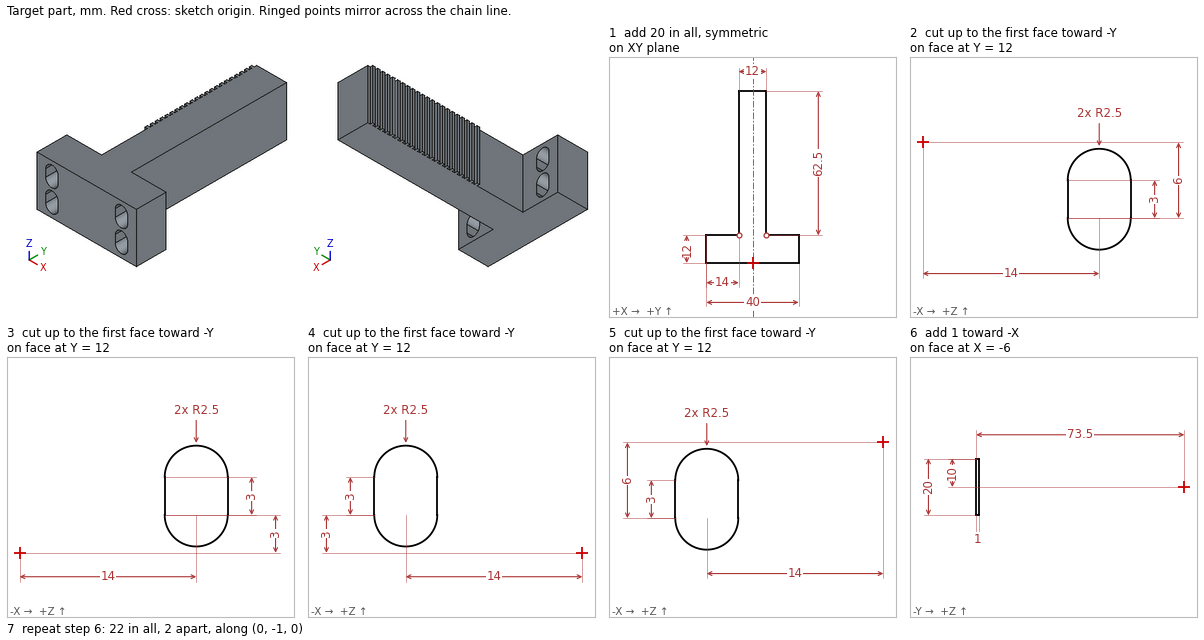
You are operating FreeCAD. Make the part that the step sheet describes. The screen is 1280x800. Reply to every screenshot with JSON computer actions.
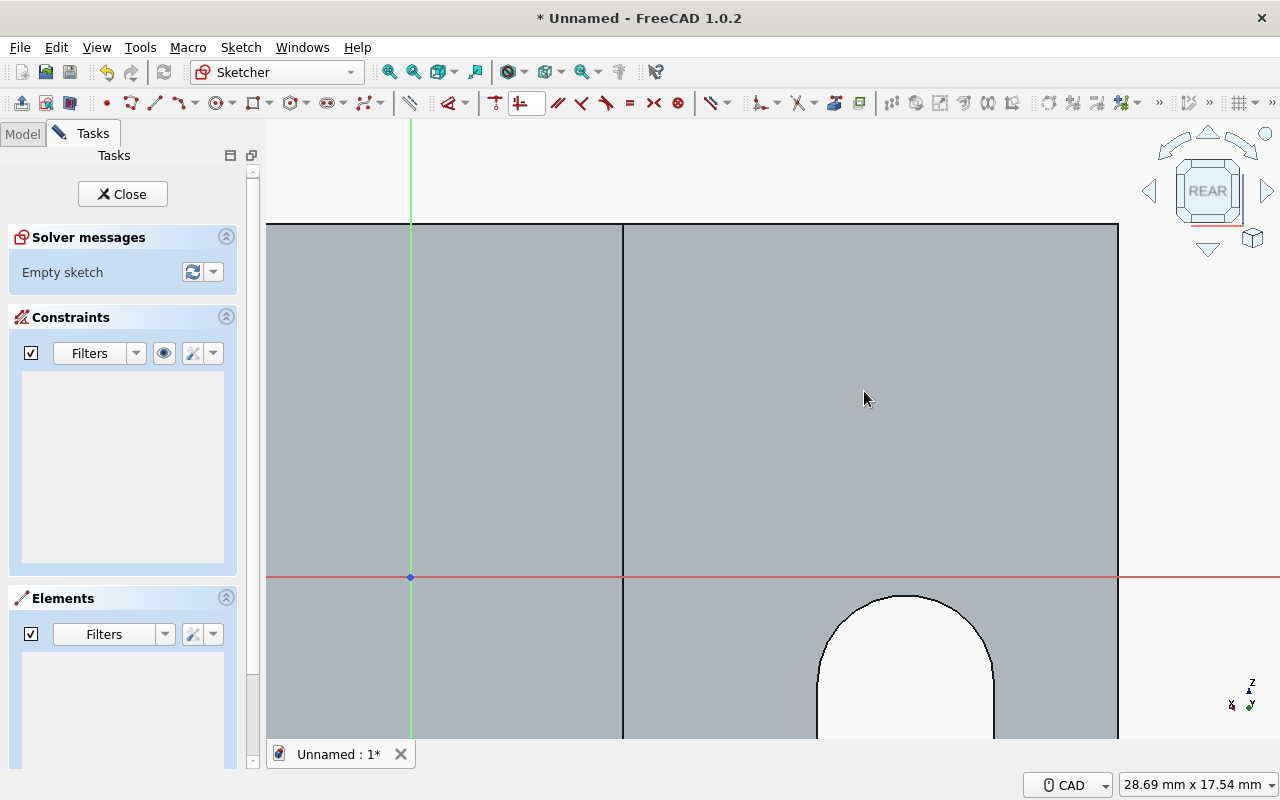
{"action": "left_click", "coordinate": [328, 104]}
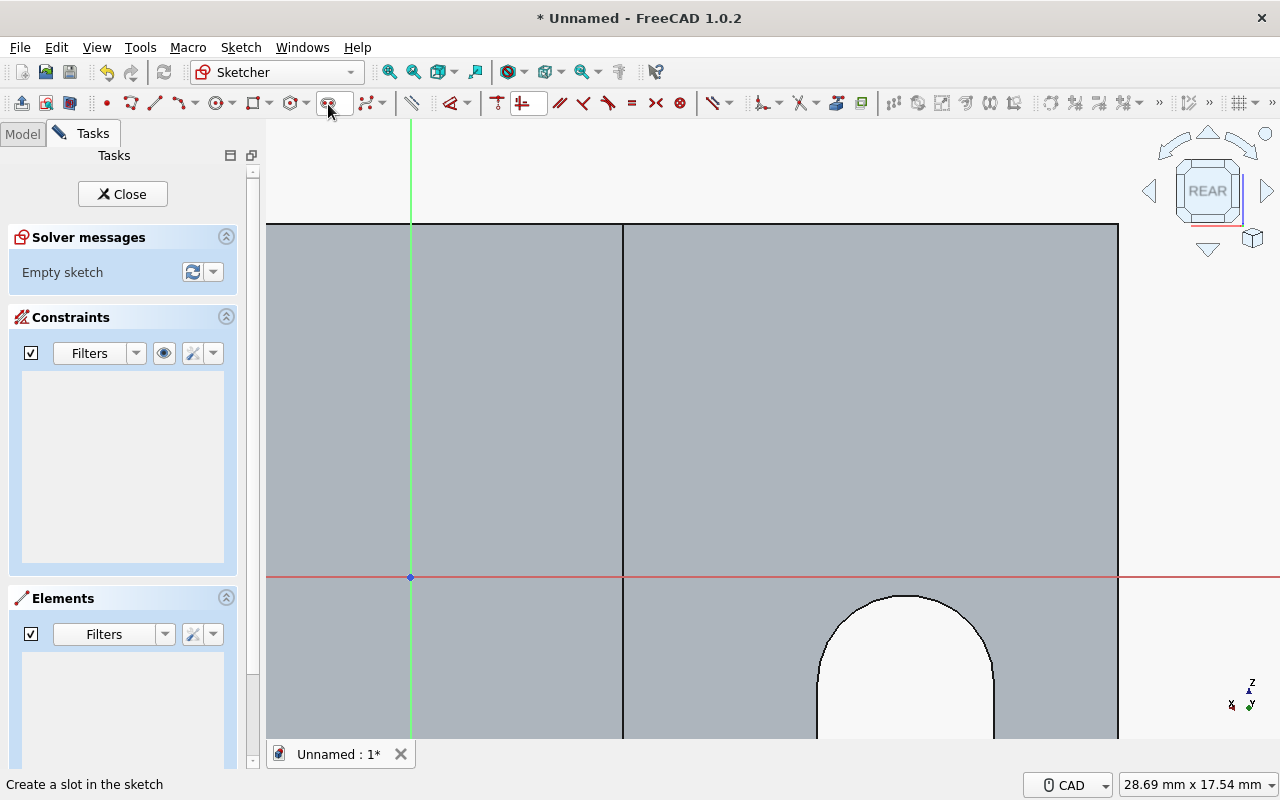
{"action": "left_click", "coordinate": [906, 471]}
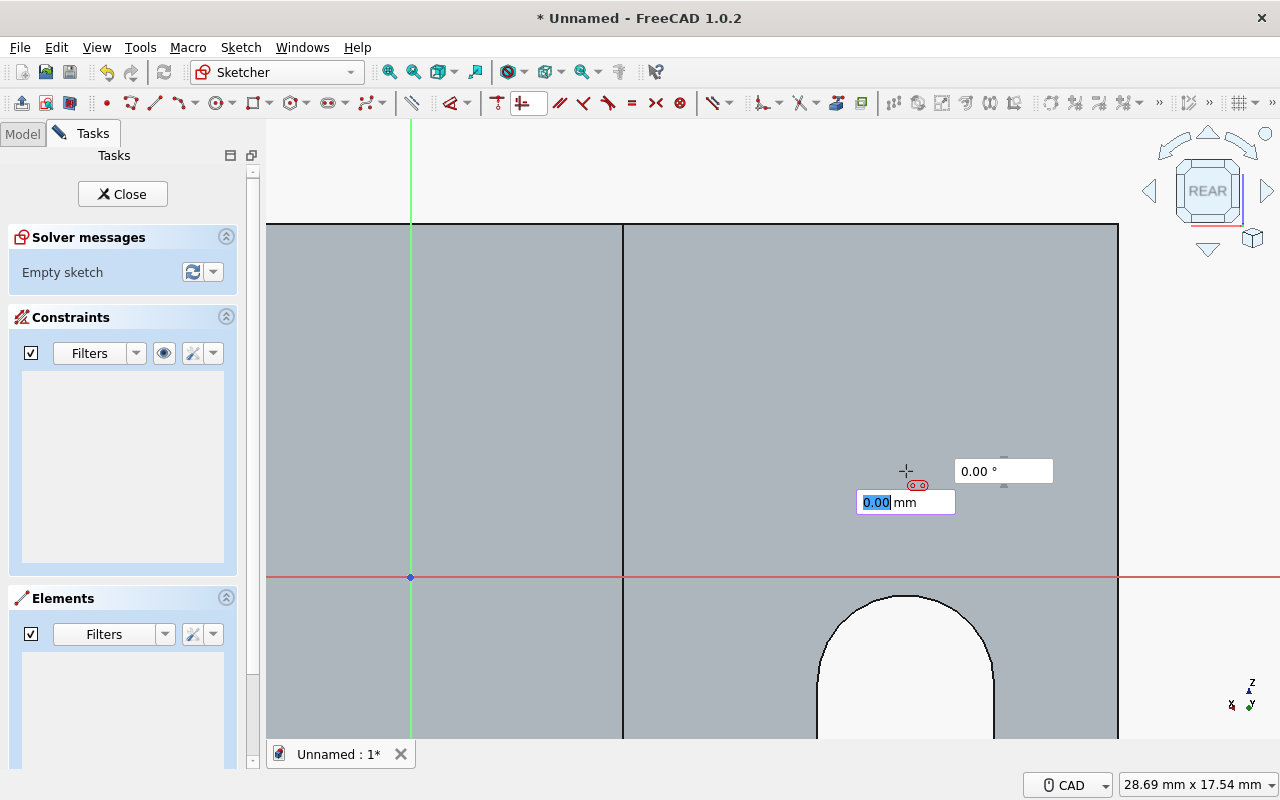
{"action": "left_click", "coordinate": [906, 365]}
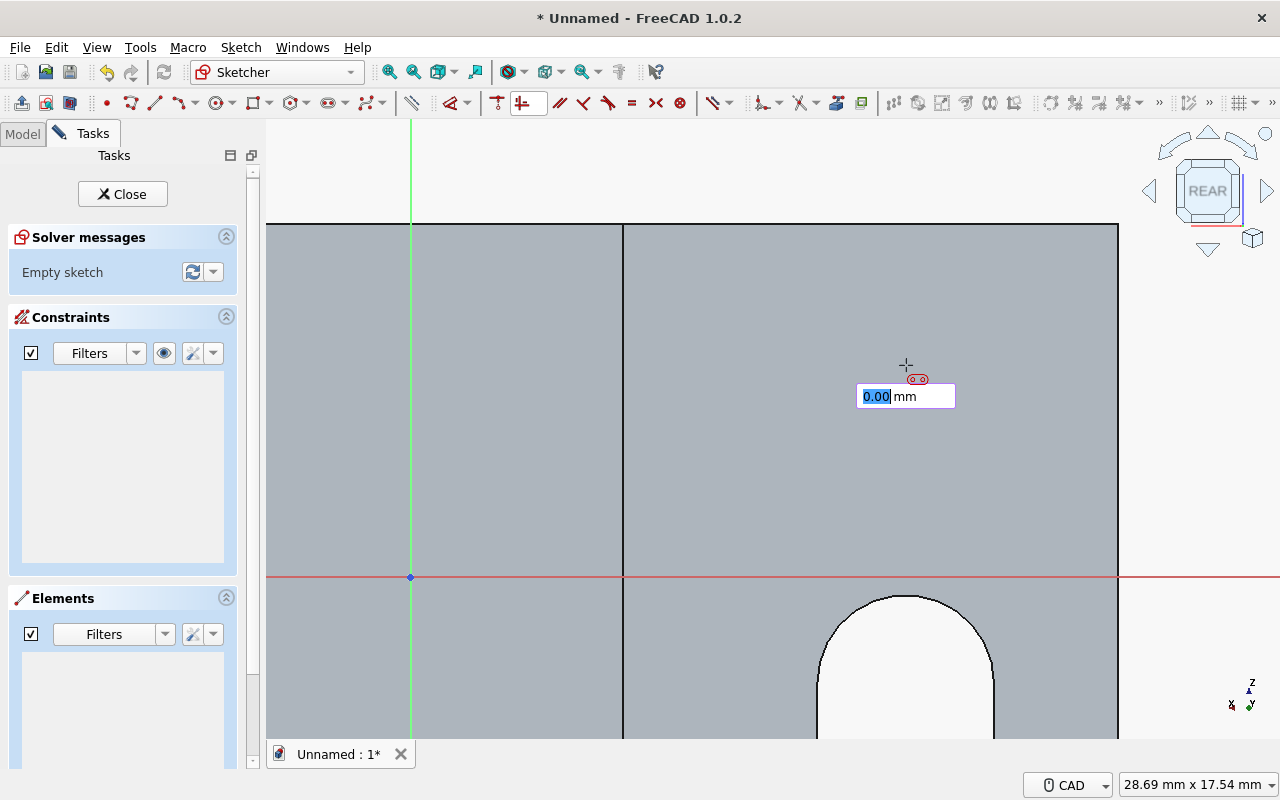
{"action": "left_click", "coordinate": [994, 418]}
{"action": "key", "text": "Escape"}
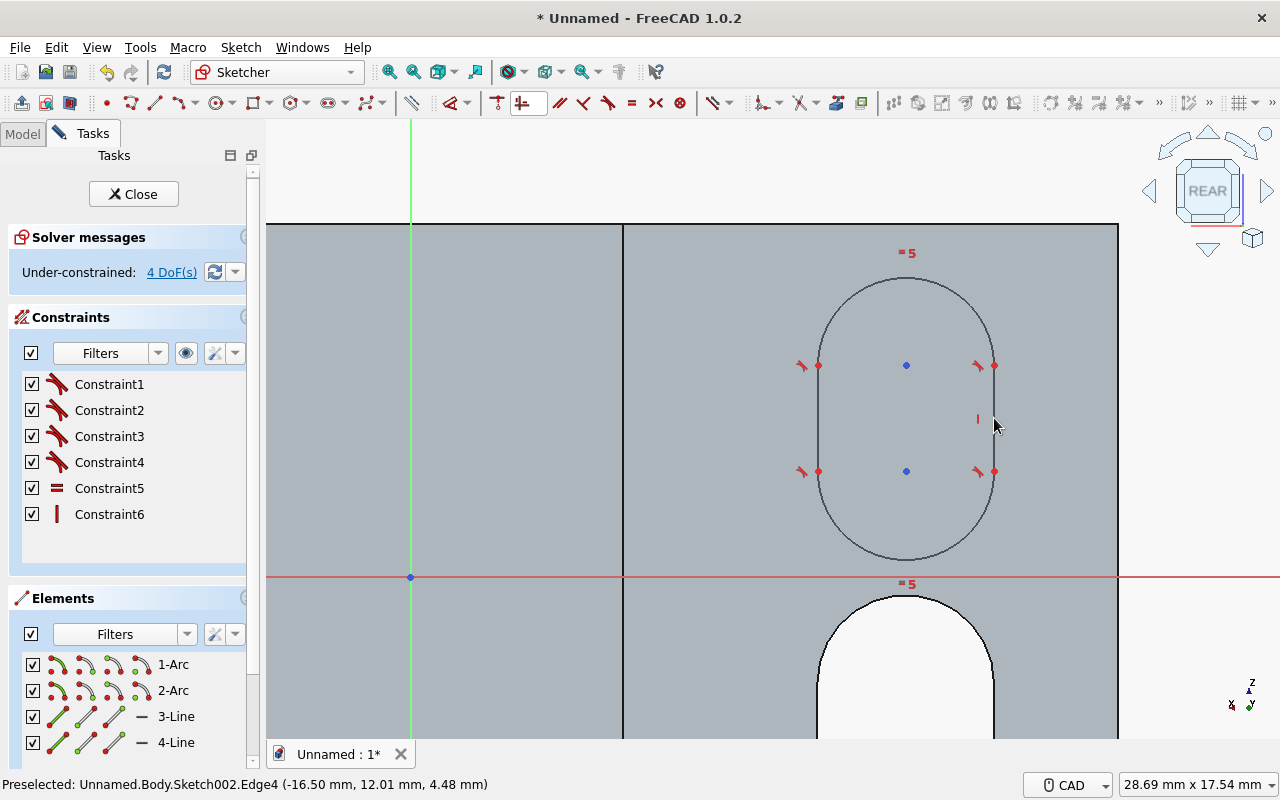
{"action": "left_click", "coordinate": [450, 104]}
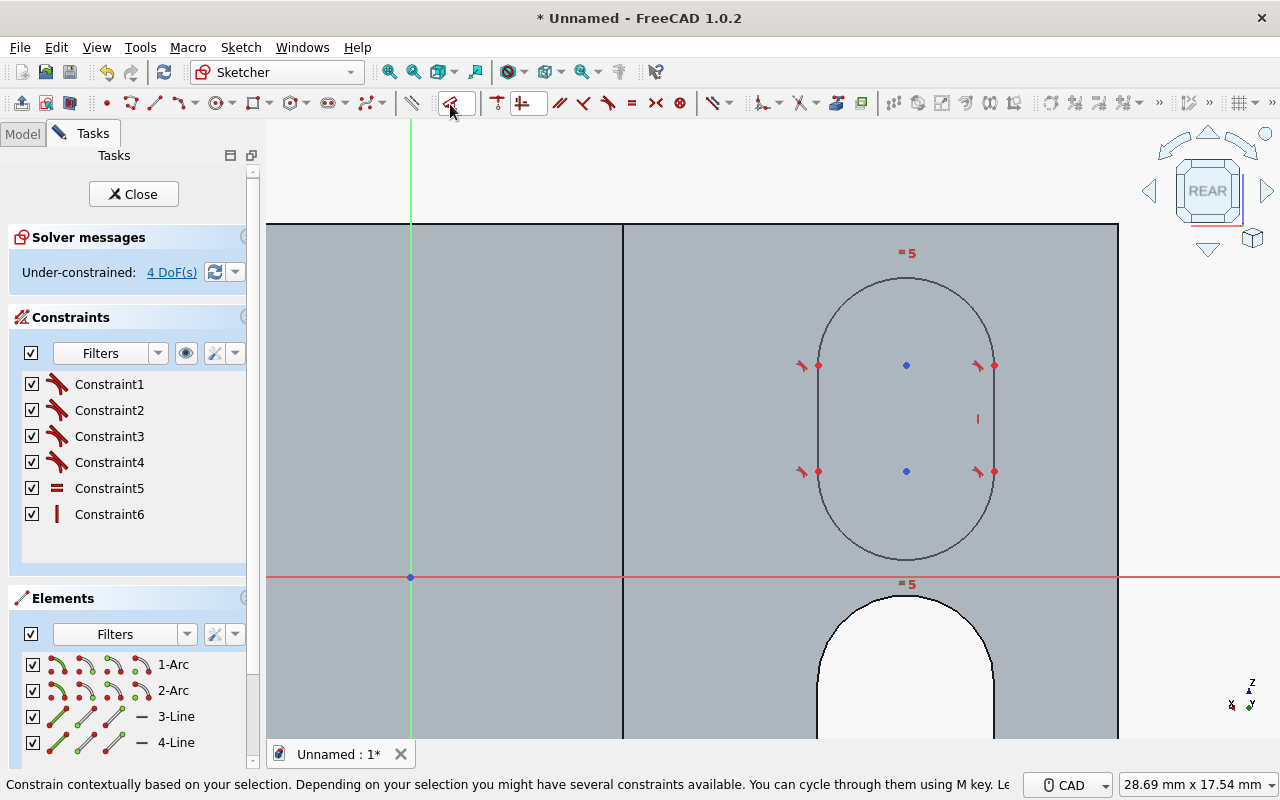
{"action": "left_click", "coordinate": [854, 543]}
{"action": "left_click", "coordinate": [797, 523]}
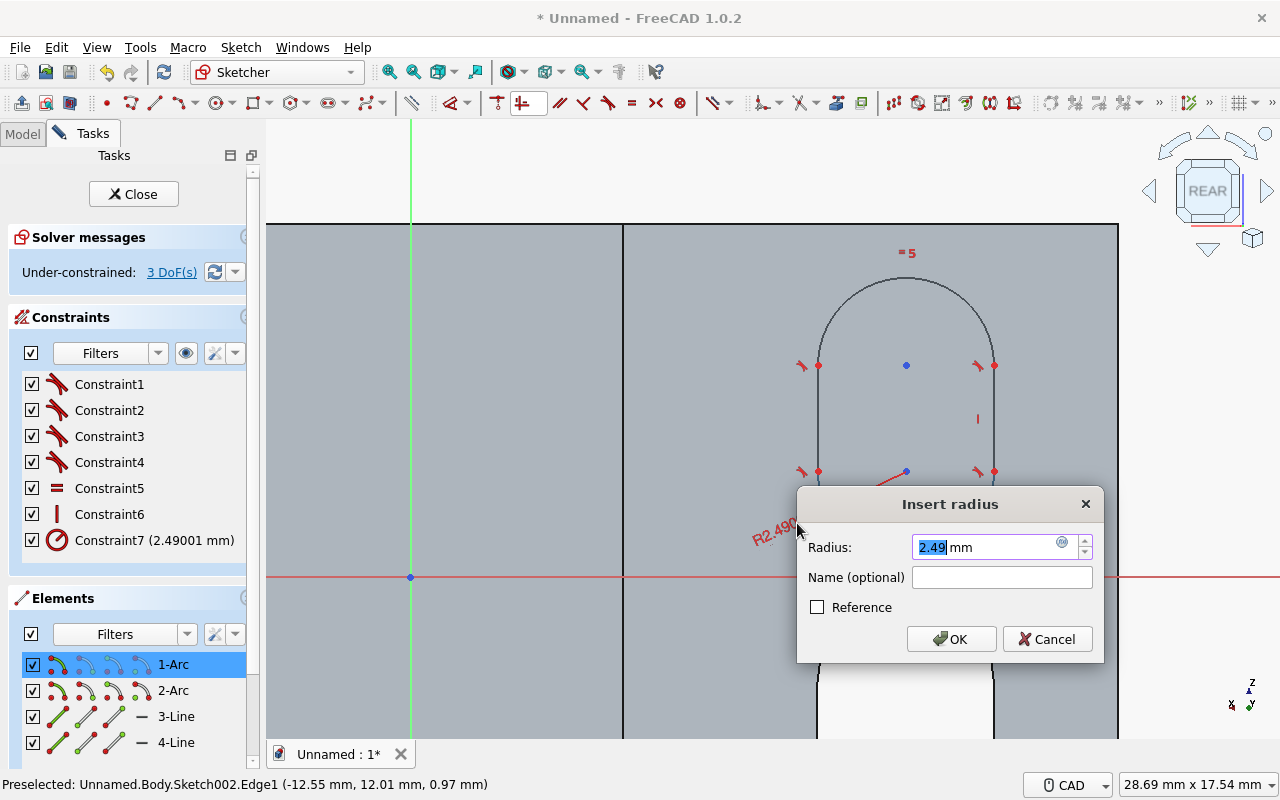
{"action": "type", "text": "2.5"}
{"action": "key", "text": "Return"}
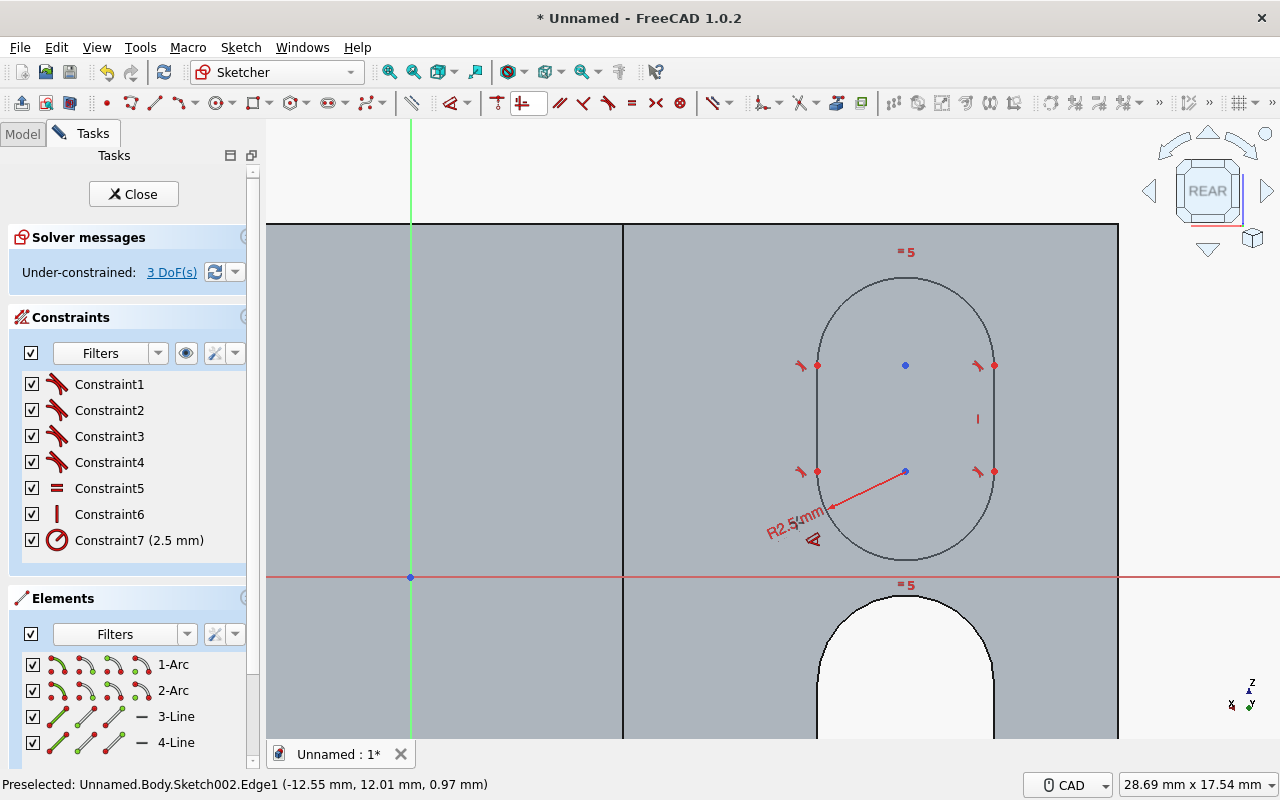
{"action": "left_click", "coordinate": [817, 440]}
{"action": "left_click", "coordinate": [851, 419]}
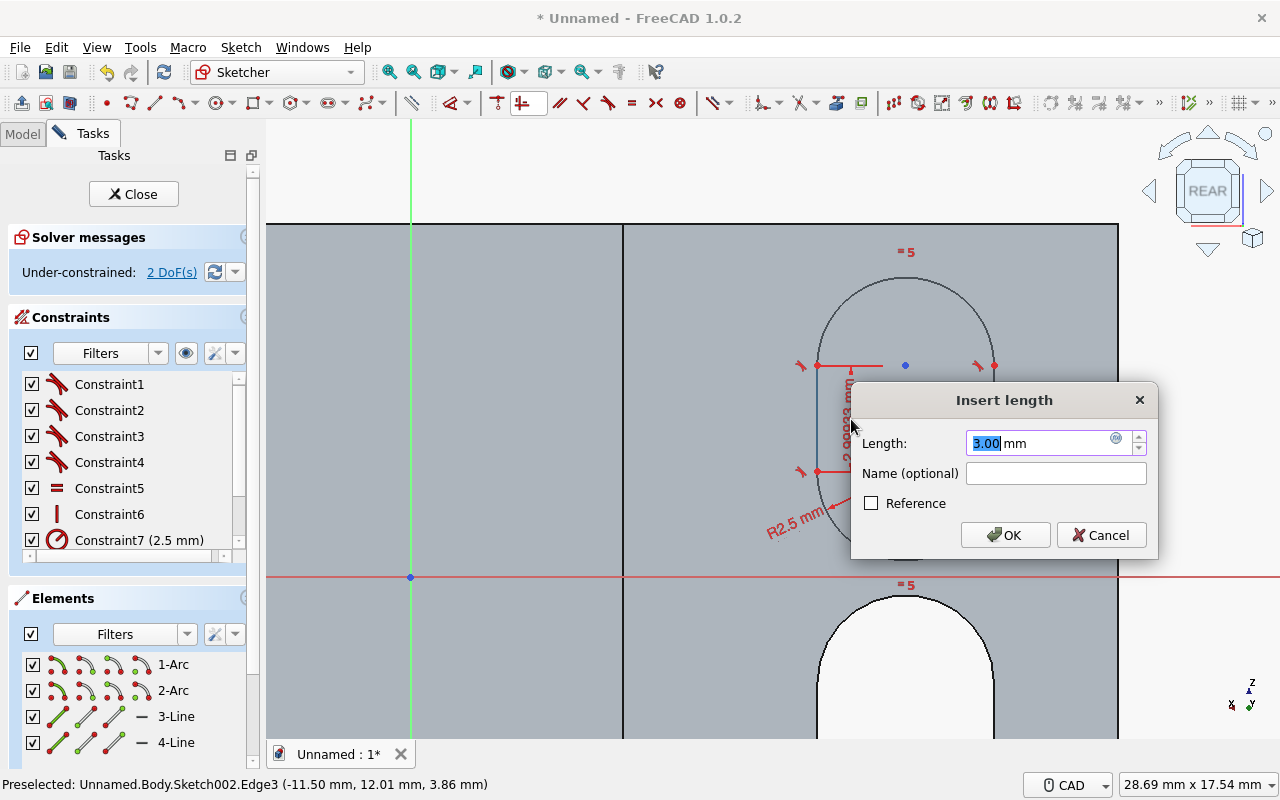
{"action": "type", "text": "3"}
{"action": "key", "text": "Return"}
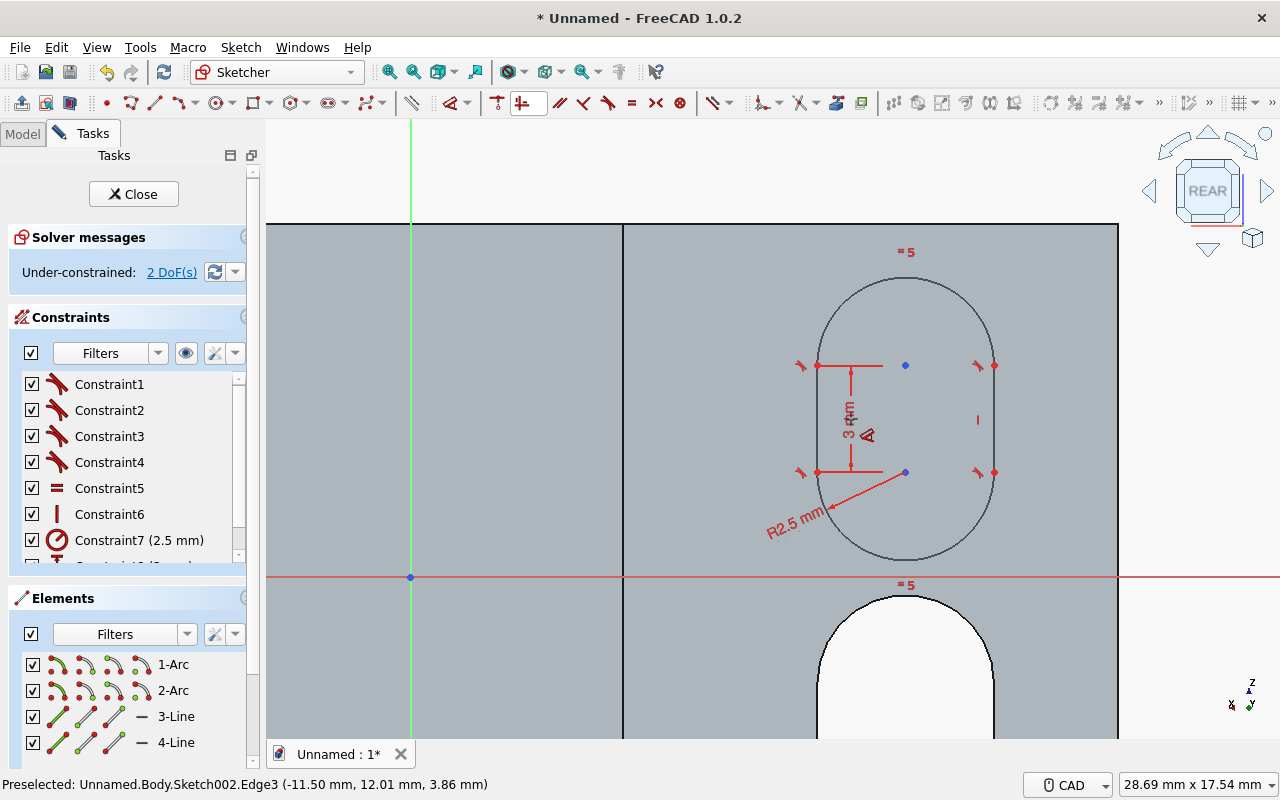
{"action": "left_click", "coordinate": [817, 472]}
{"action": "left_click", "coordinate": [377, 525]}